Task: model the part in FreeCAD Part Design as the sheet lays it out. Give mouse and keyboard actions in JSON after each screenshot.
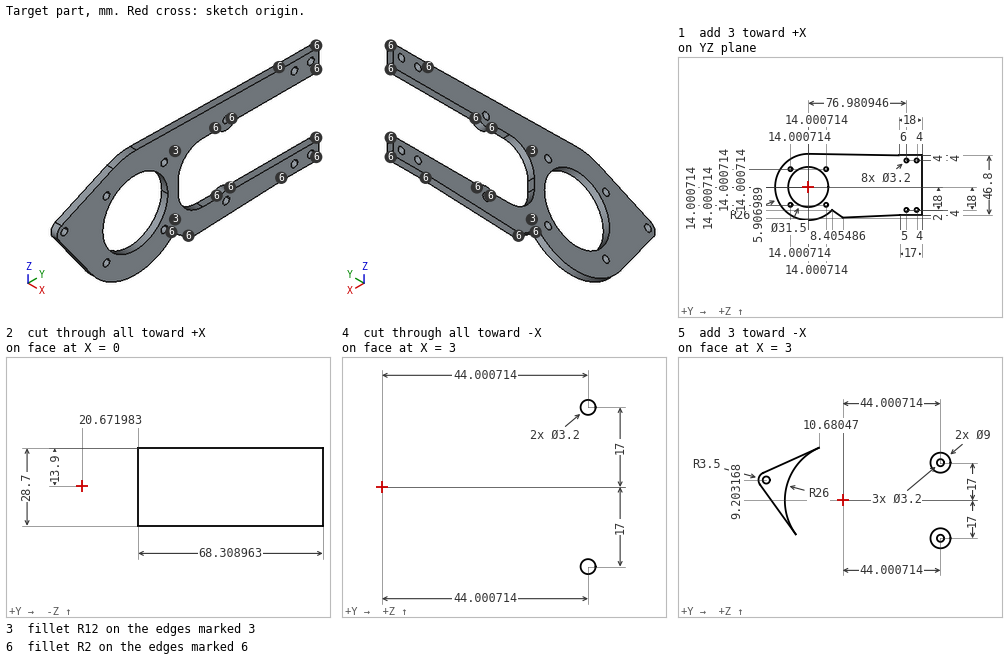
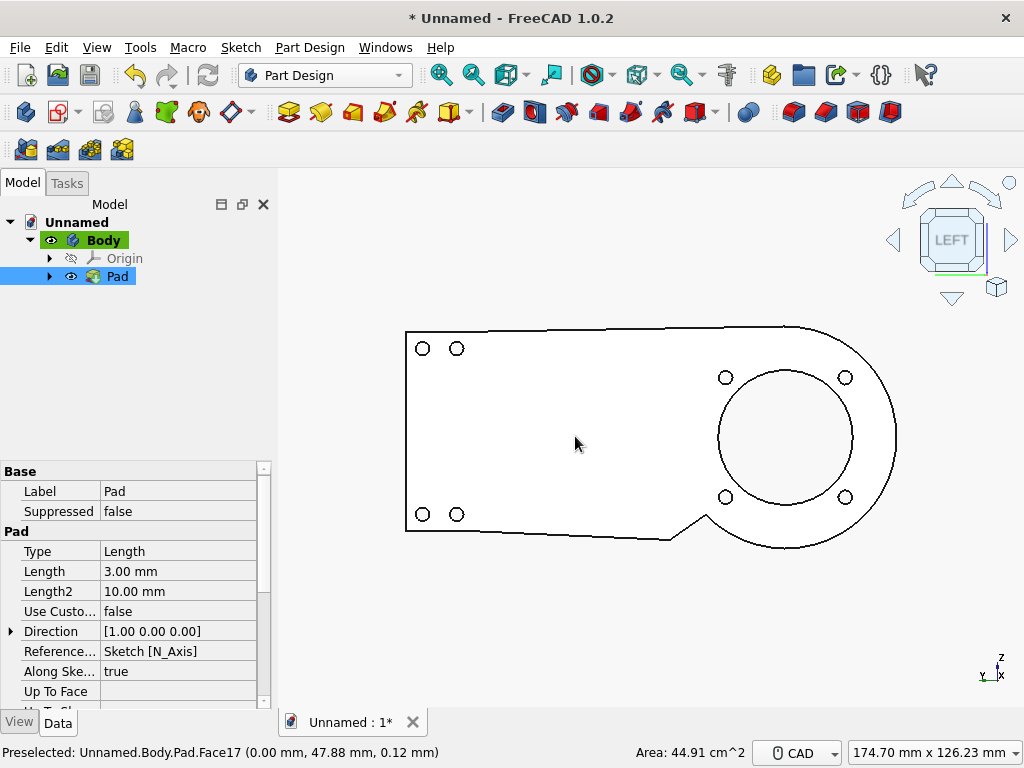
{"action": "left_click", "coordinate": [58, 112]}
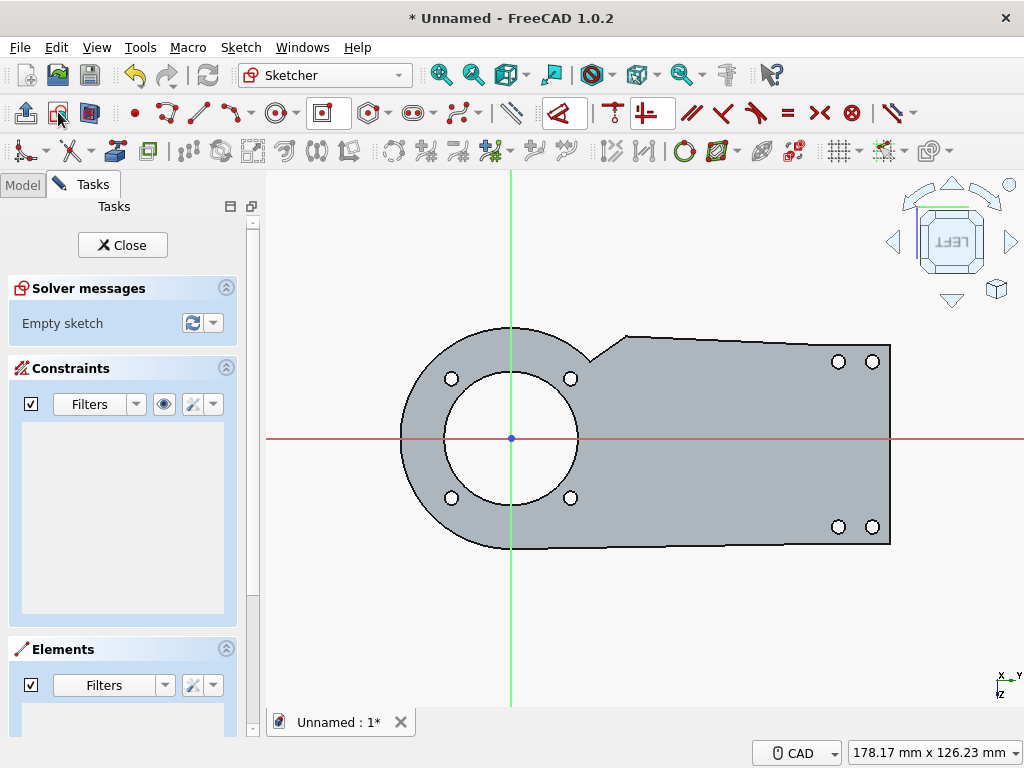
{"action": "scroll", "coordinate": [294, 430], "scroll_direction": "down", "scroll_amount": 1}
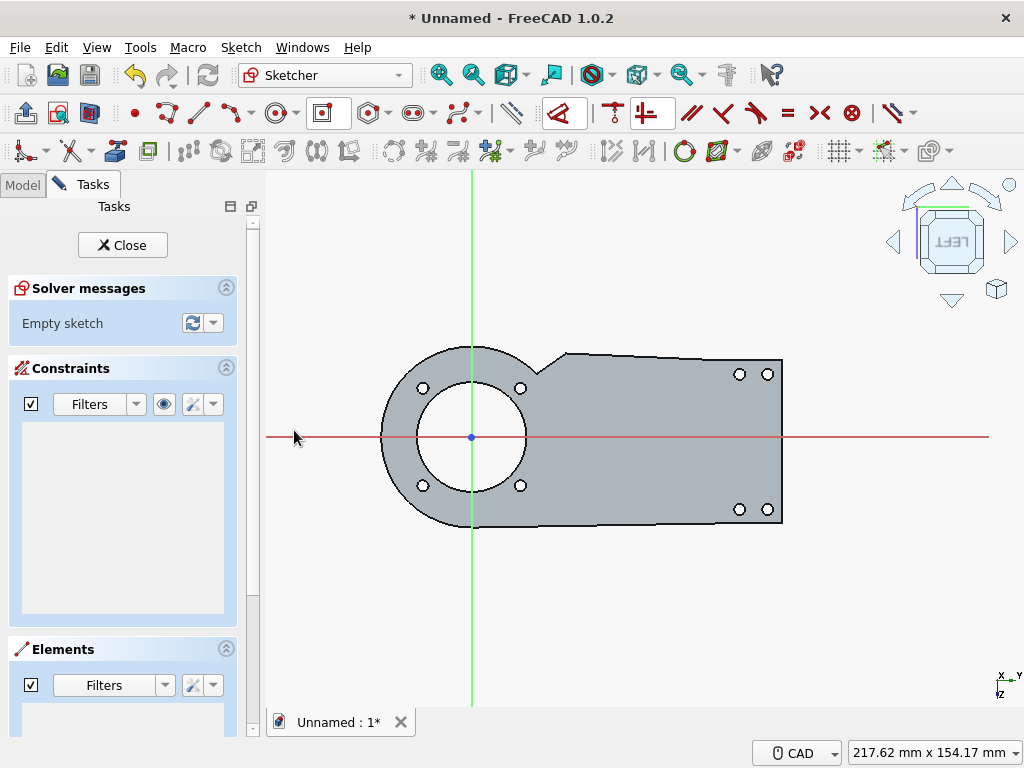
{"action": "left_click", "coordinate": [346, 114]}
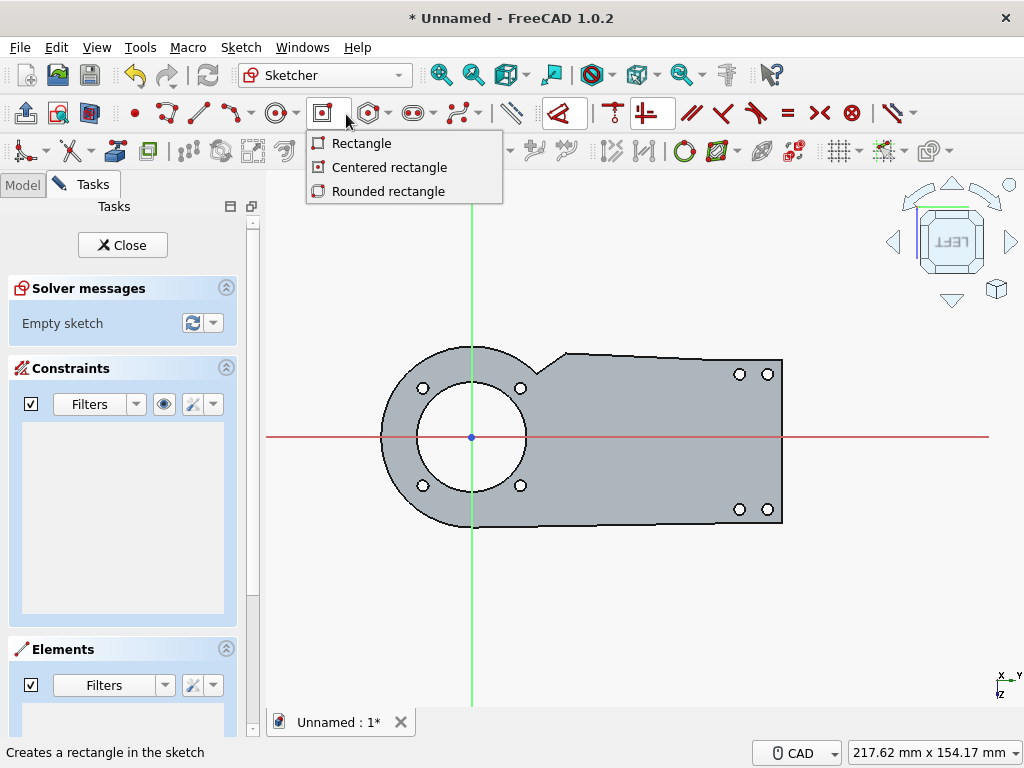
{"action": "left_click", "coordinate": [404, 143]}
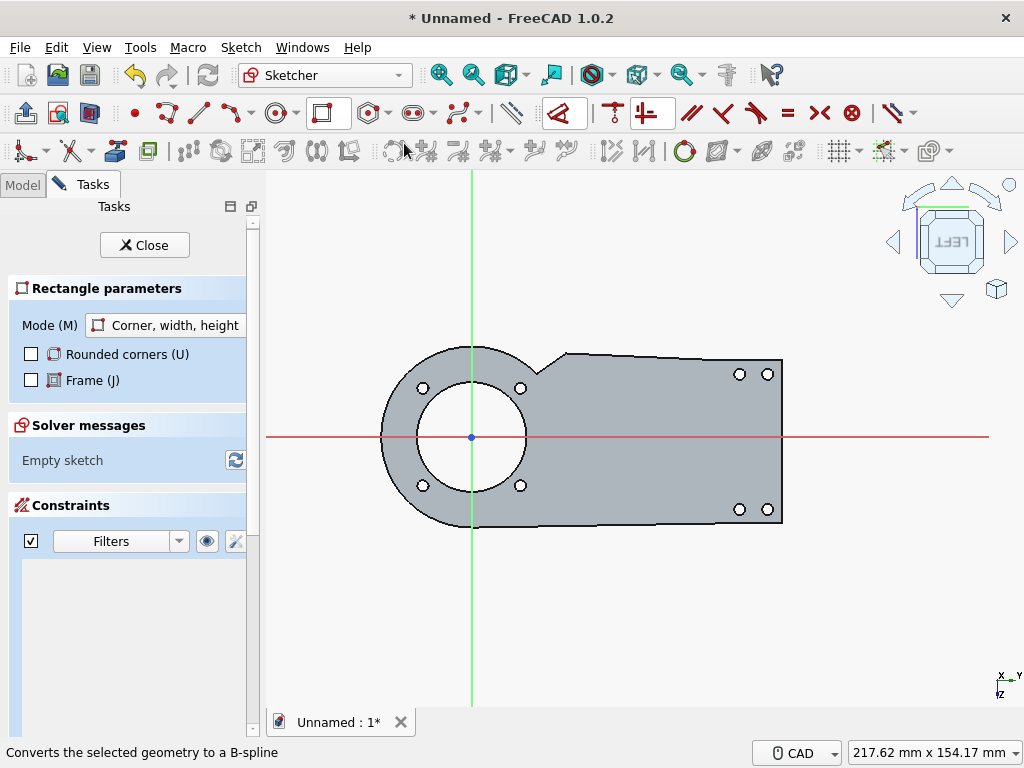
{"action": "left_click", "coordinate": [544, 389]}
{"action": "left_click", "coordinate": [782, 489]}
{"action": "key", "text": "Escape"}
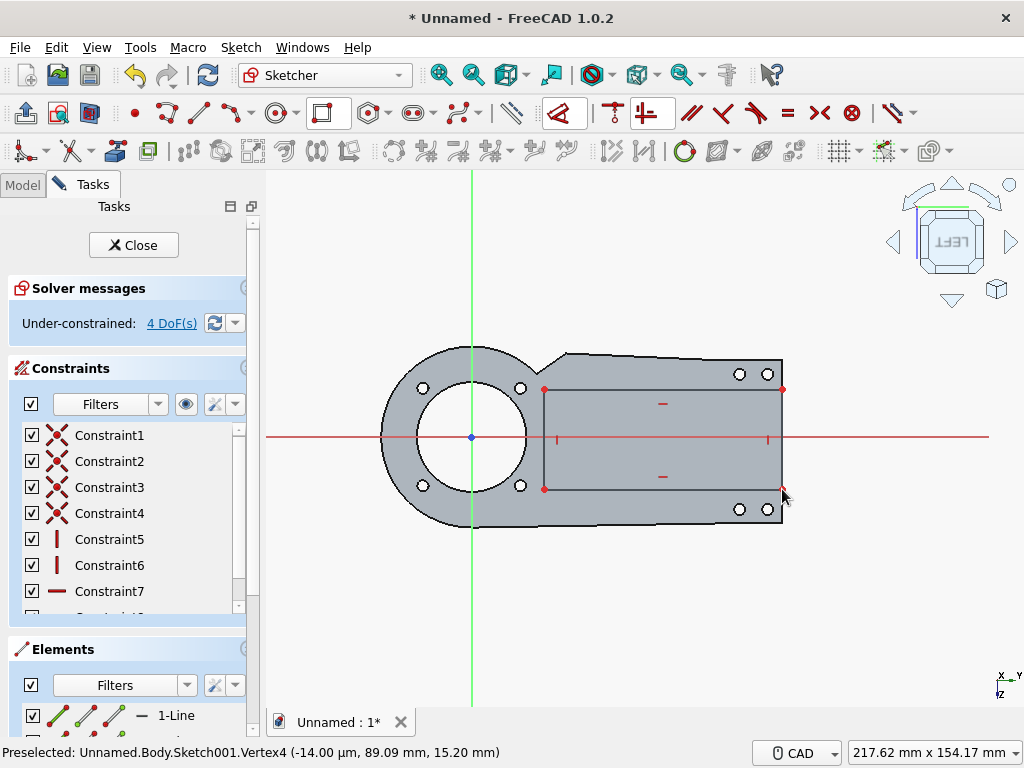
{"action": "left_click", "coordinate": [544, 420]}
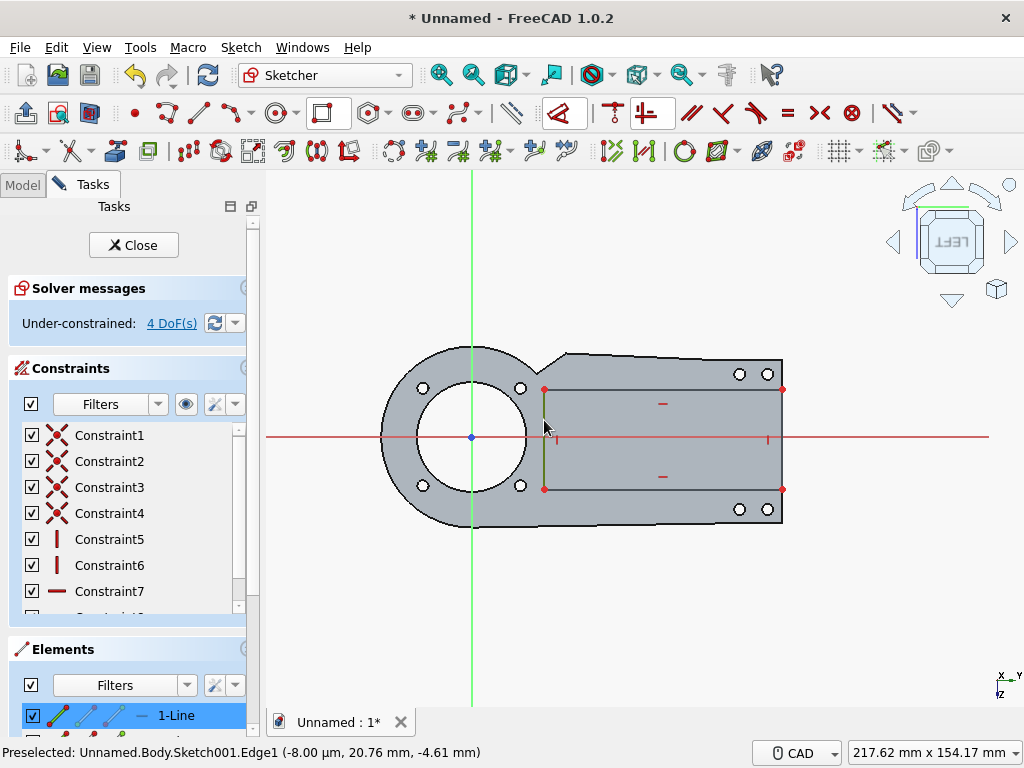
{"action": "left_click", "coordinate": [582, 114]}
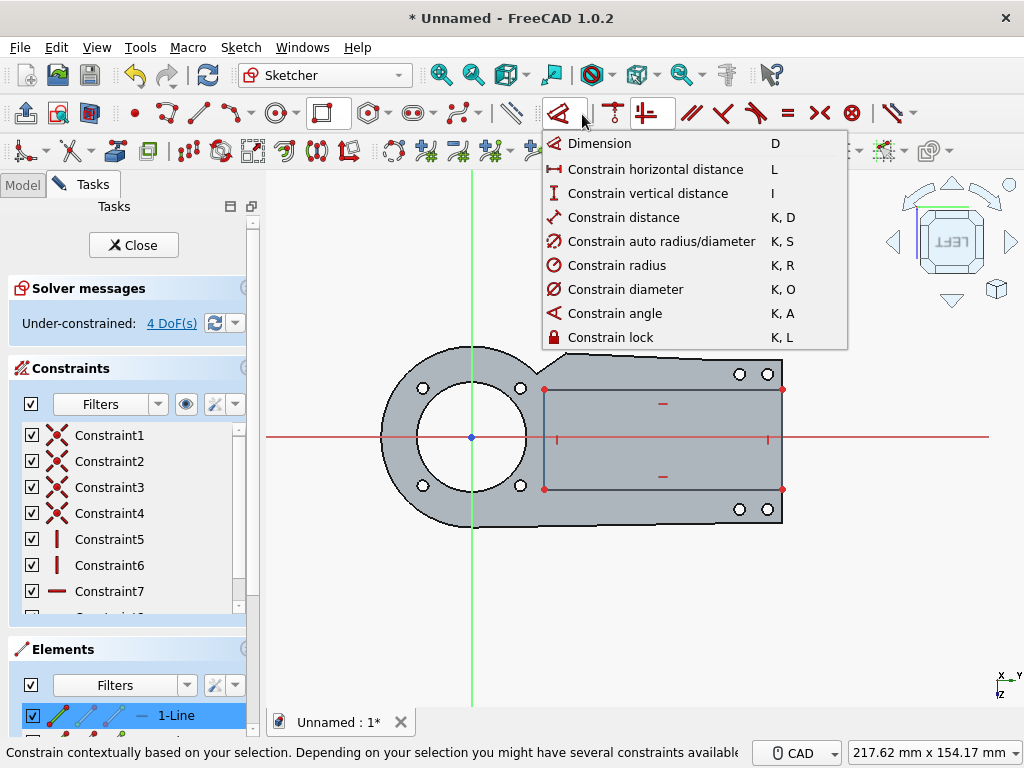
{"action": "left_click", "coordinate": [695, 193]}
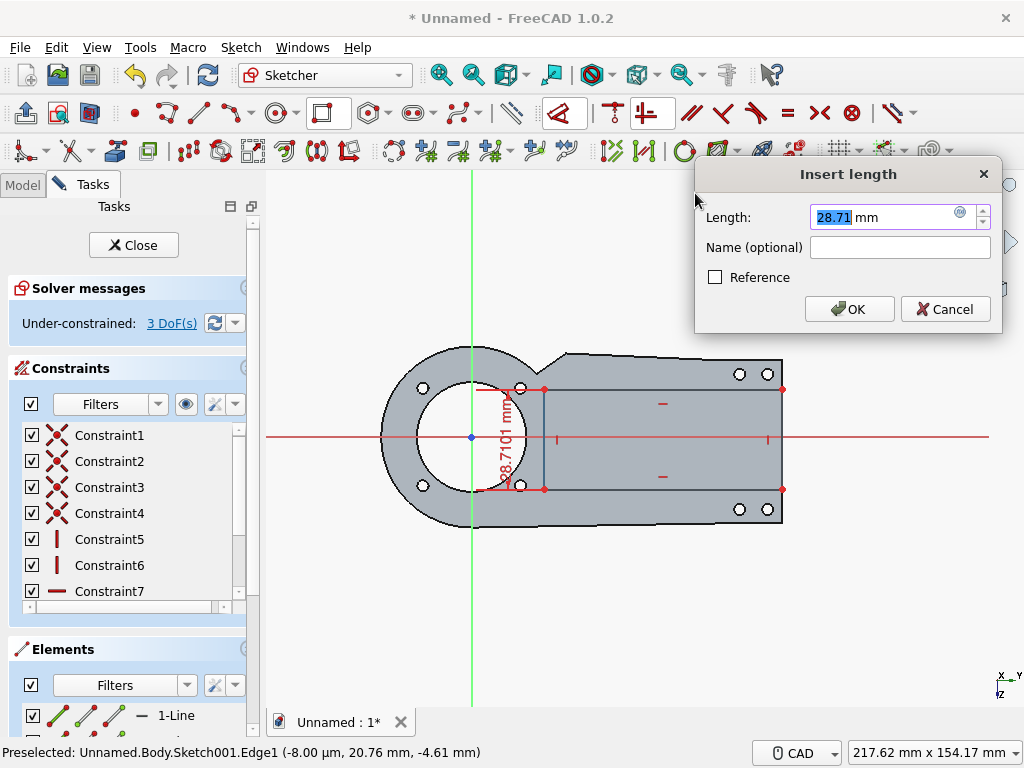
{"action": "type", "text": "28.7"}
{"action": "key", "text": "Return"}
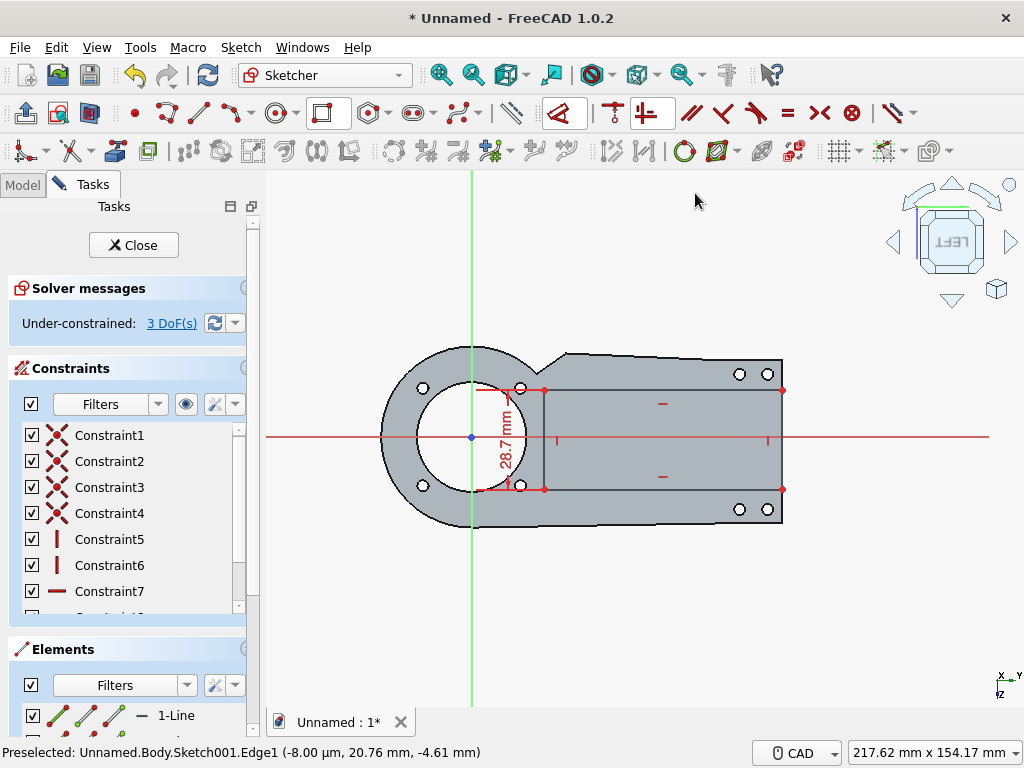
{"action": "left_click", "coordinate": [544, 390]}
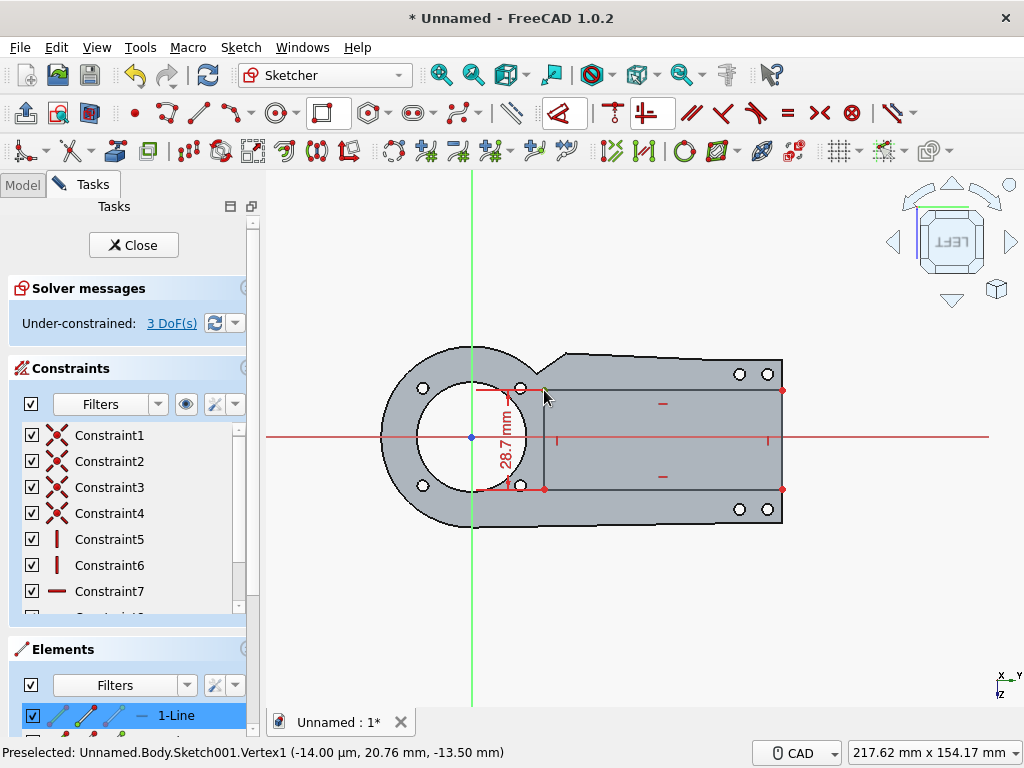
{"action": "key", "text": "i"}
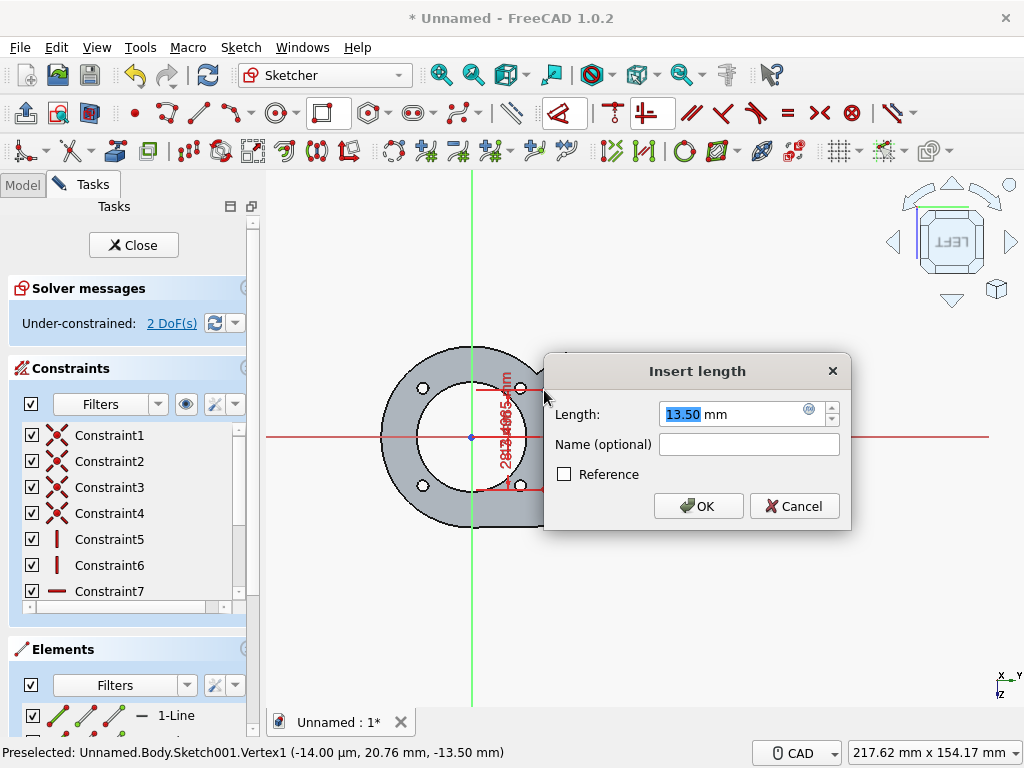
{"action": "type", "text": "13.9"}
{"action": "key", "text": "Return"}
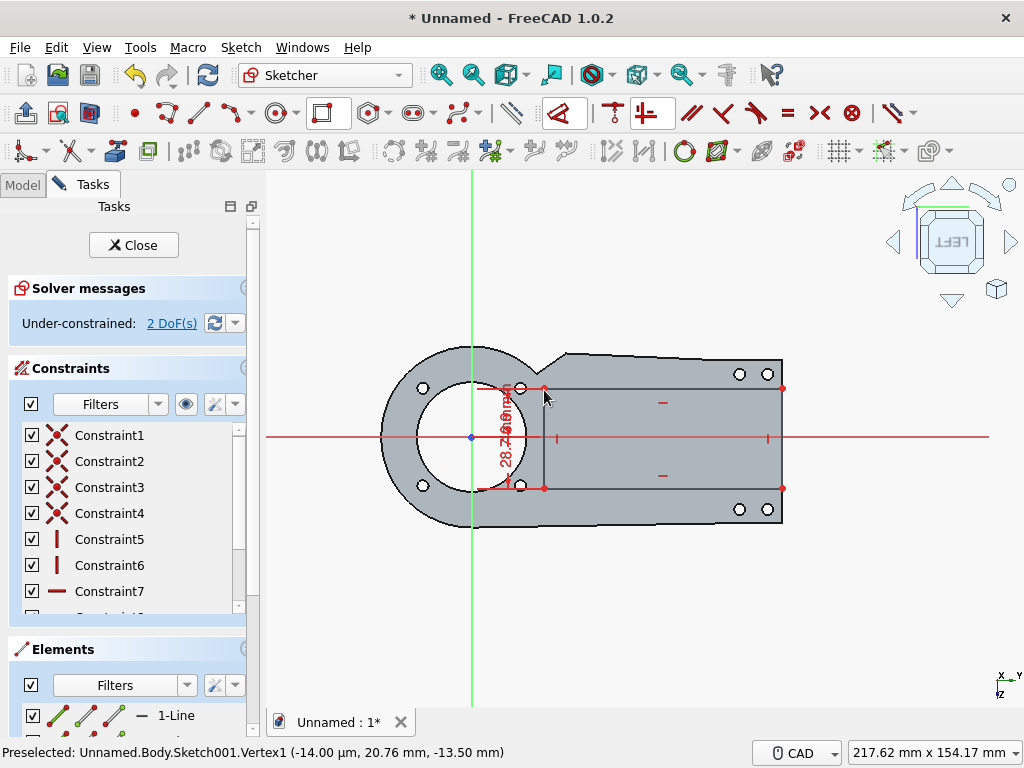
{"action": "left_click", "coordinate": [615, 489]}